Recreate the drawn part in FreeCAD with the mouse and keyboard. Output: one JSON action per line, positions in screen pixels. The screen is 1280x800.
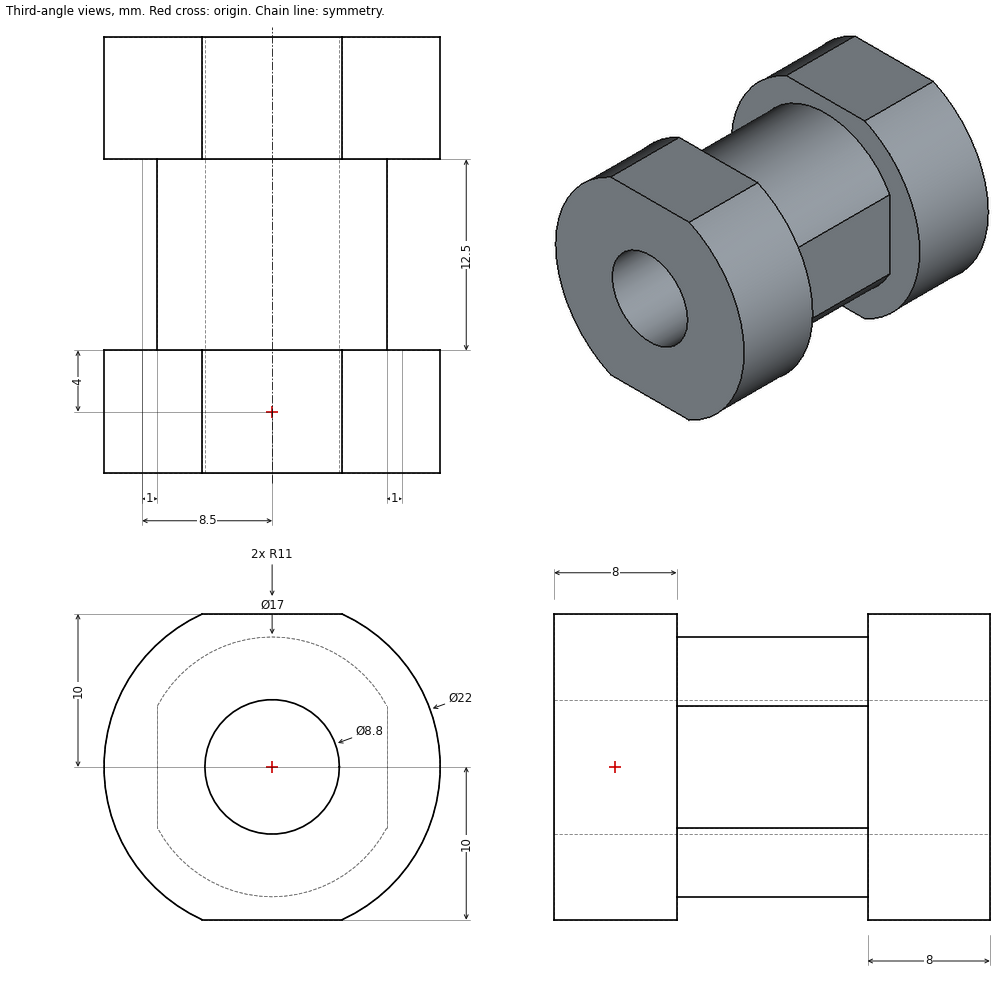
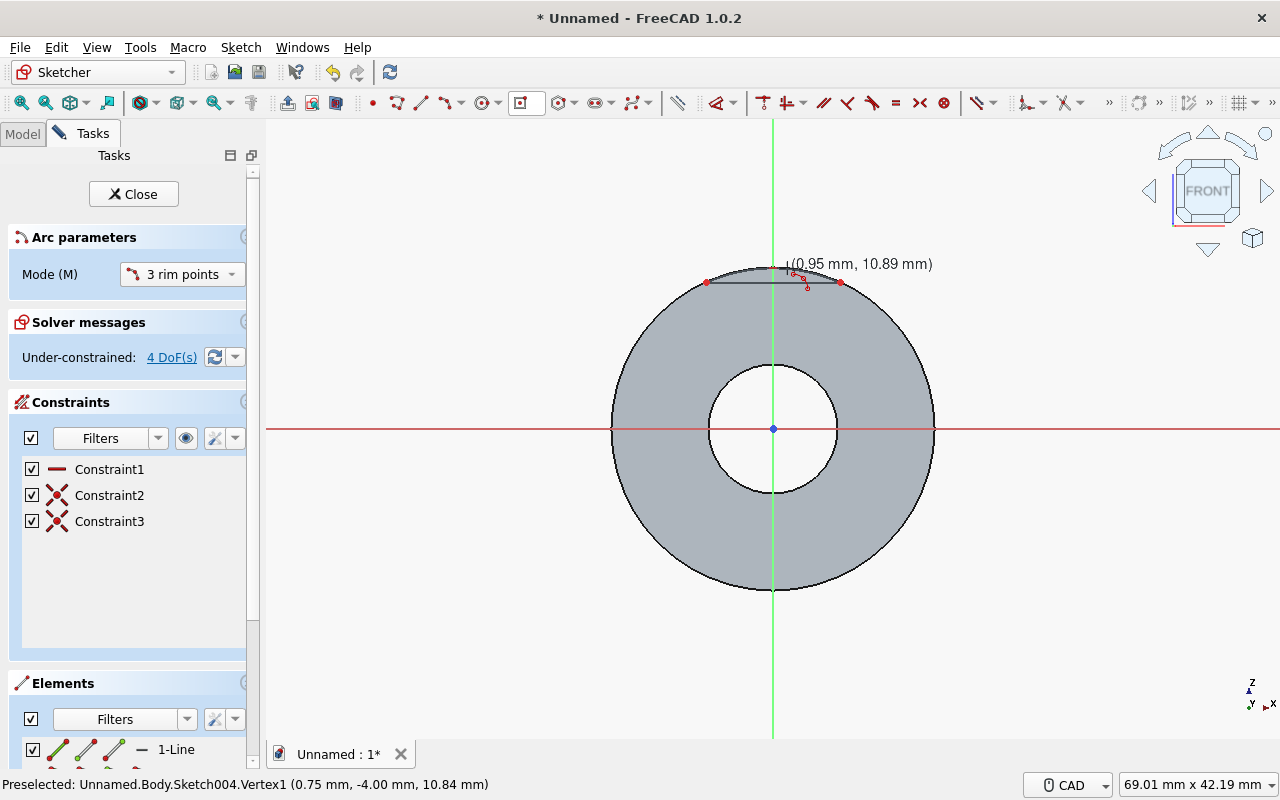
{"action": "left_click", "coordinate": [422, 104]}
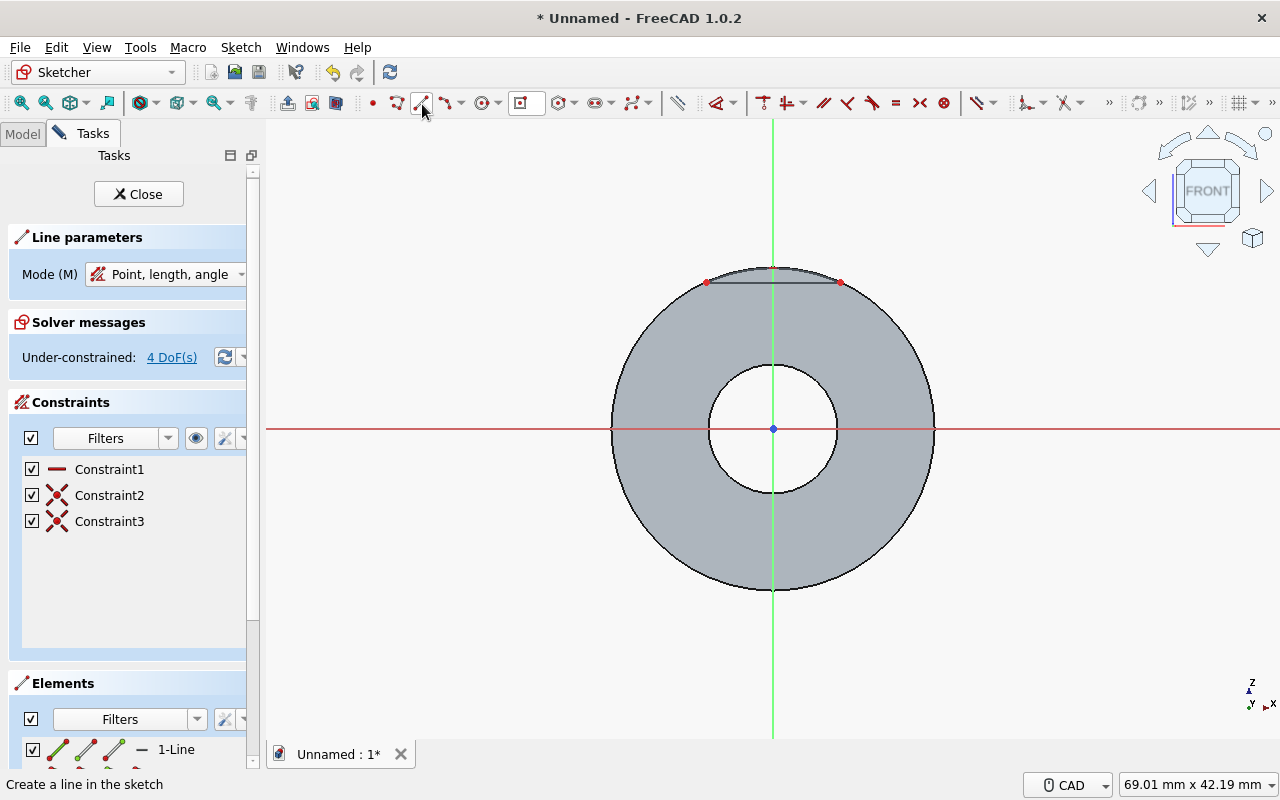
{"action": "left_click", "coordinate": [840, 576]}
{"action": "left_click", "coordinate": [706, 576]}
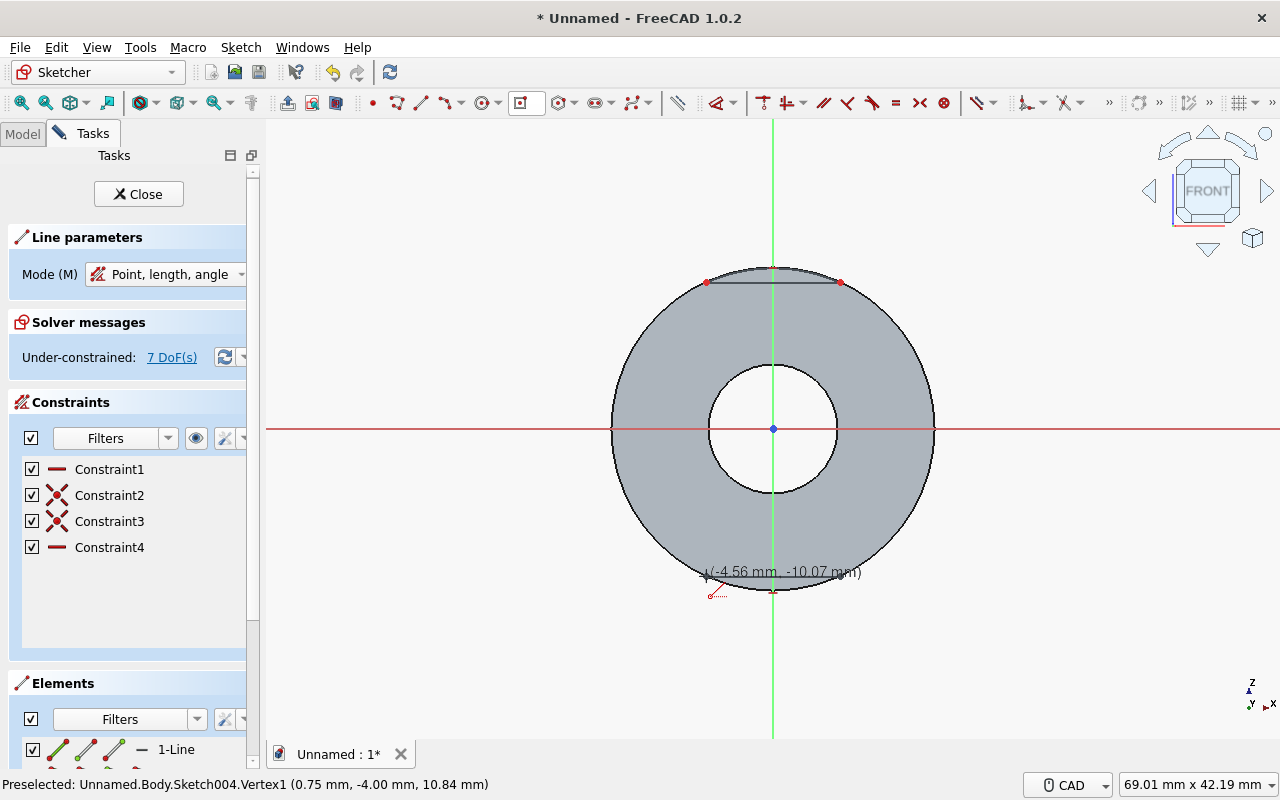
{"action": "left_click", "coordinate": [446, 104]}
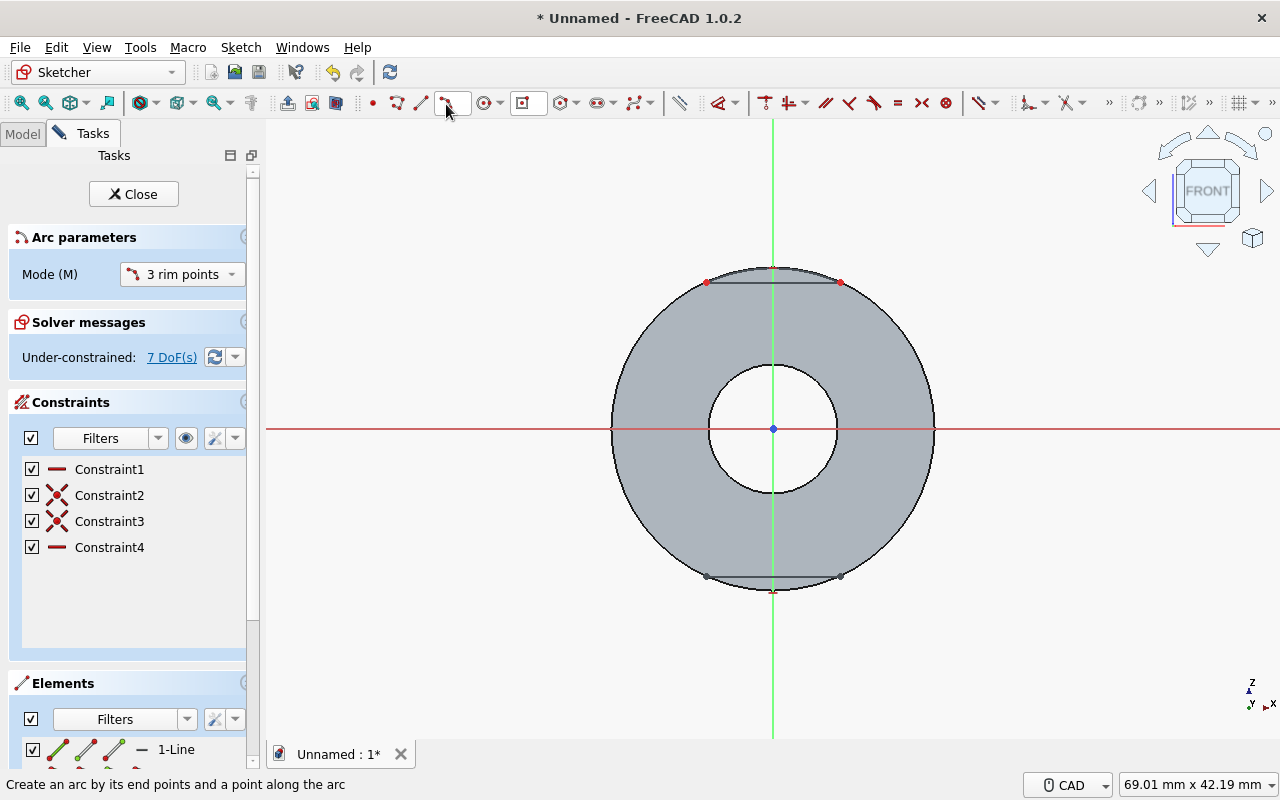
{"action": "left_click", "coordinate": [706, 577]}
{"action": "left_click", "coordinate": [840, 577]}
{"action": "left_click", "coordinate": [787, 590]}
{"action": "key", "text": "Escape"}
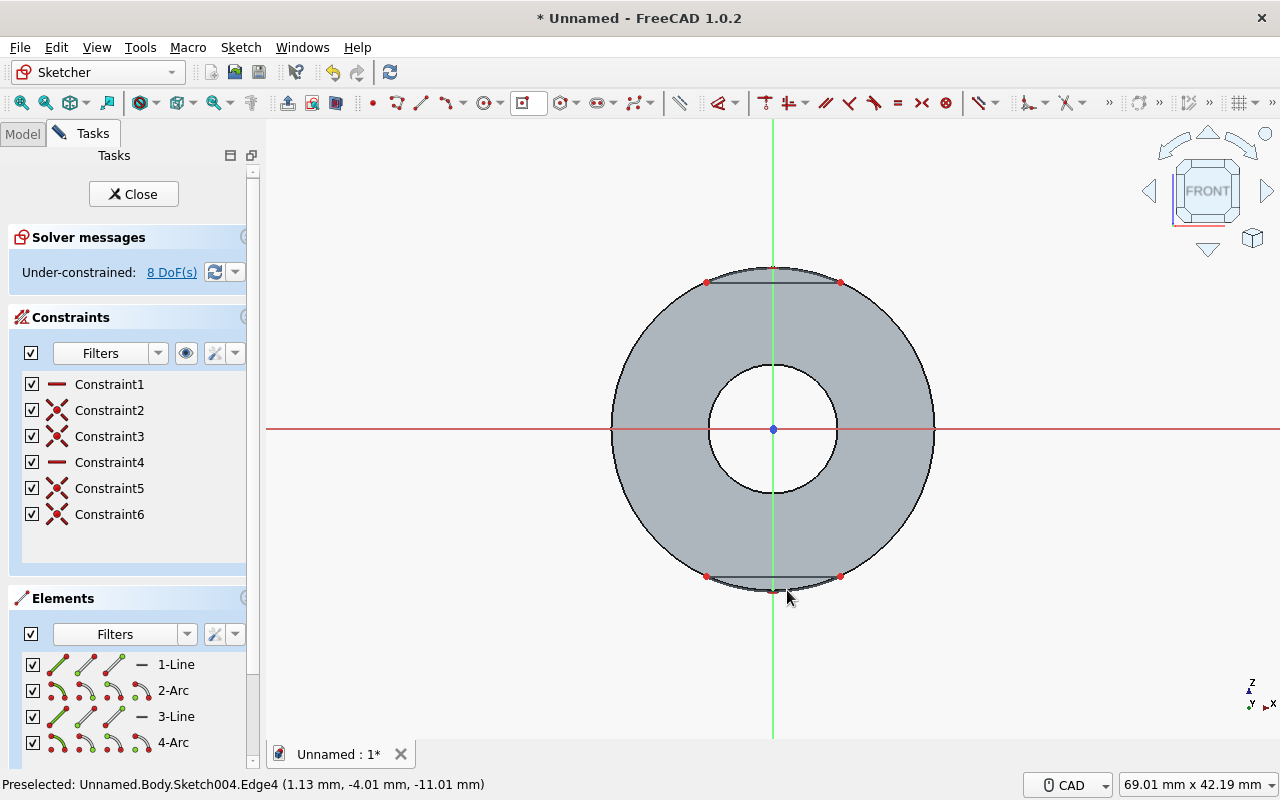
{"action": "left_click", "coordinate": [801, 271]}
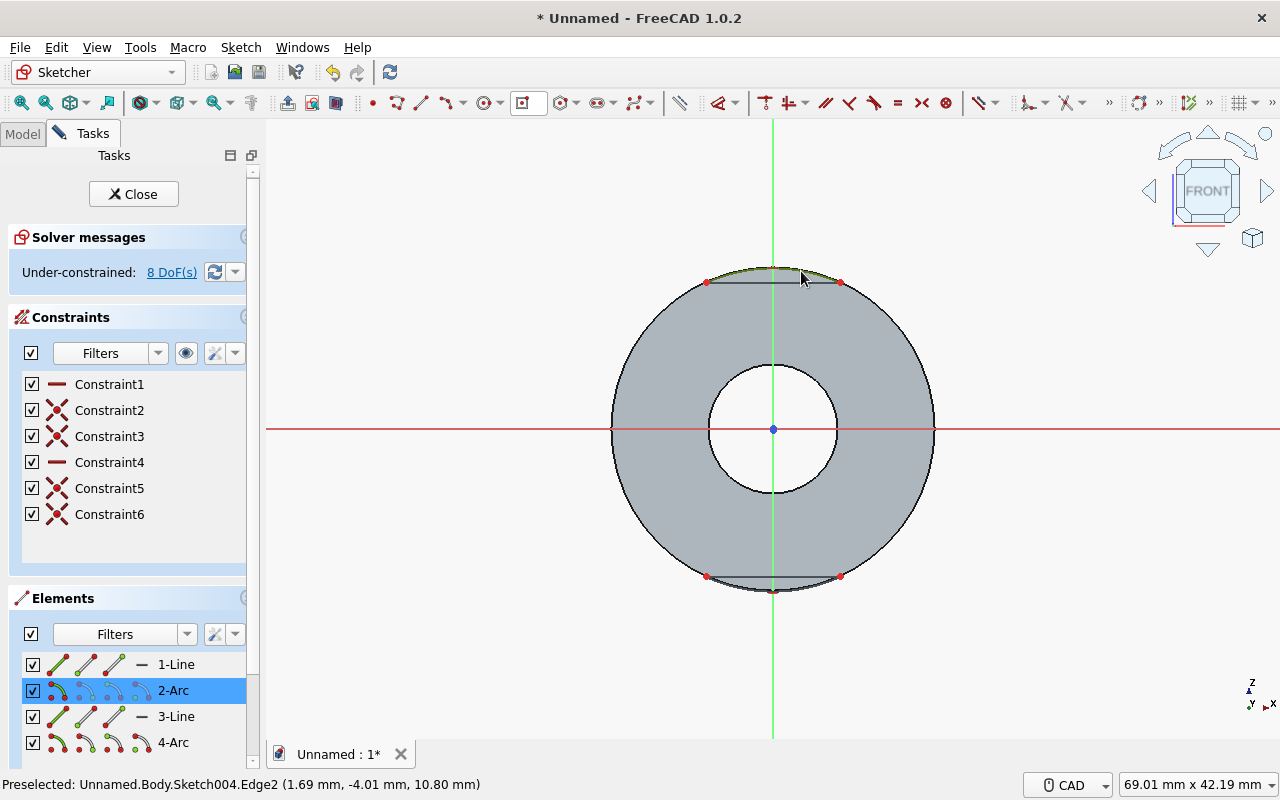
{"action": "left_click", "coordinate": [745, 589]}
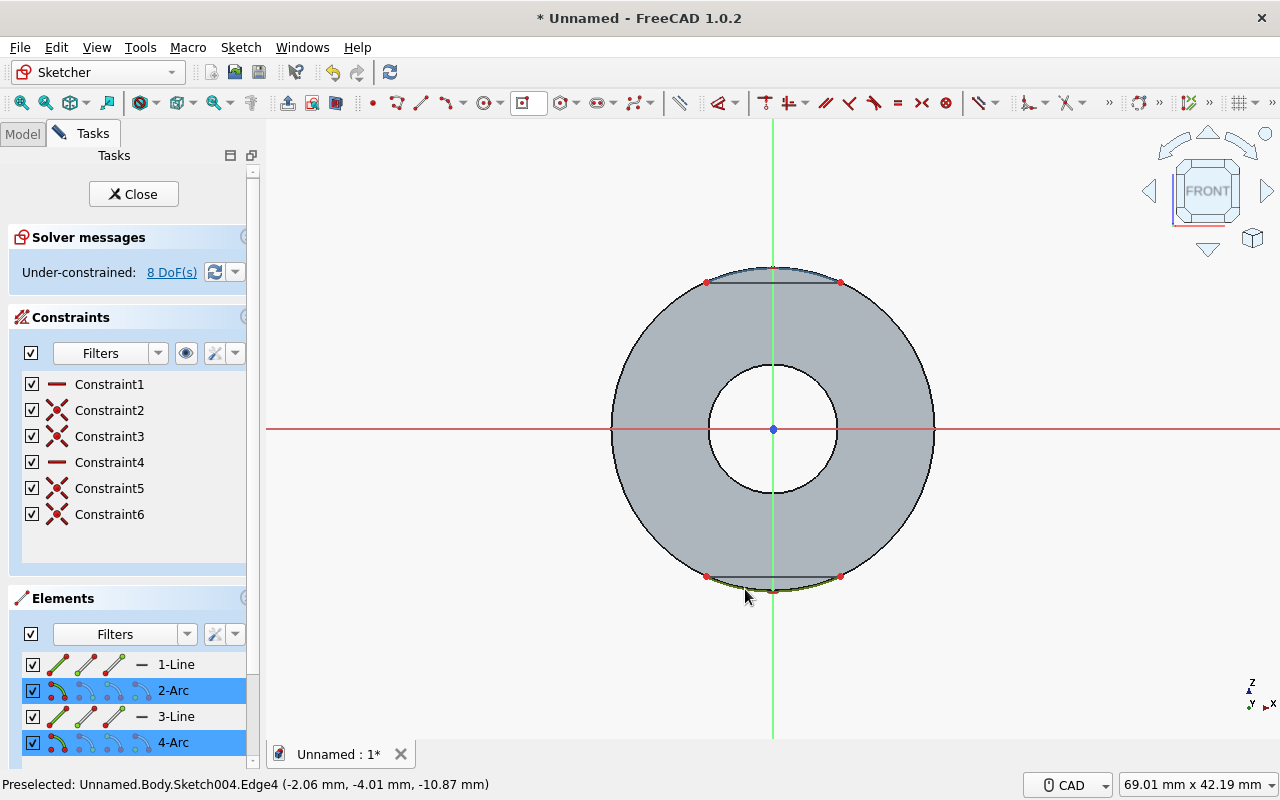
{"action": "left_click", "coordinate": [766, 104]}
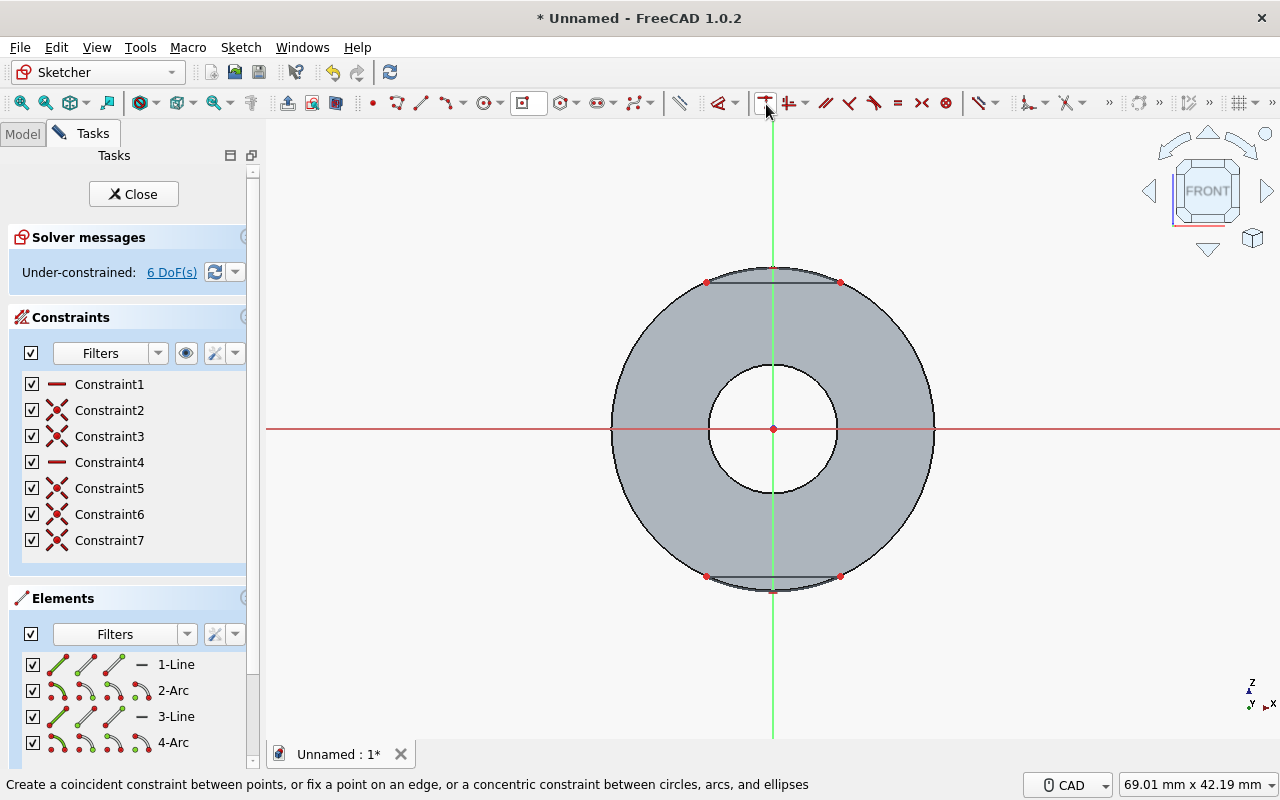
{"action": "left_click_drag", "start_coordinate": [763, 419], "coordinate": [783, 439]}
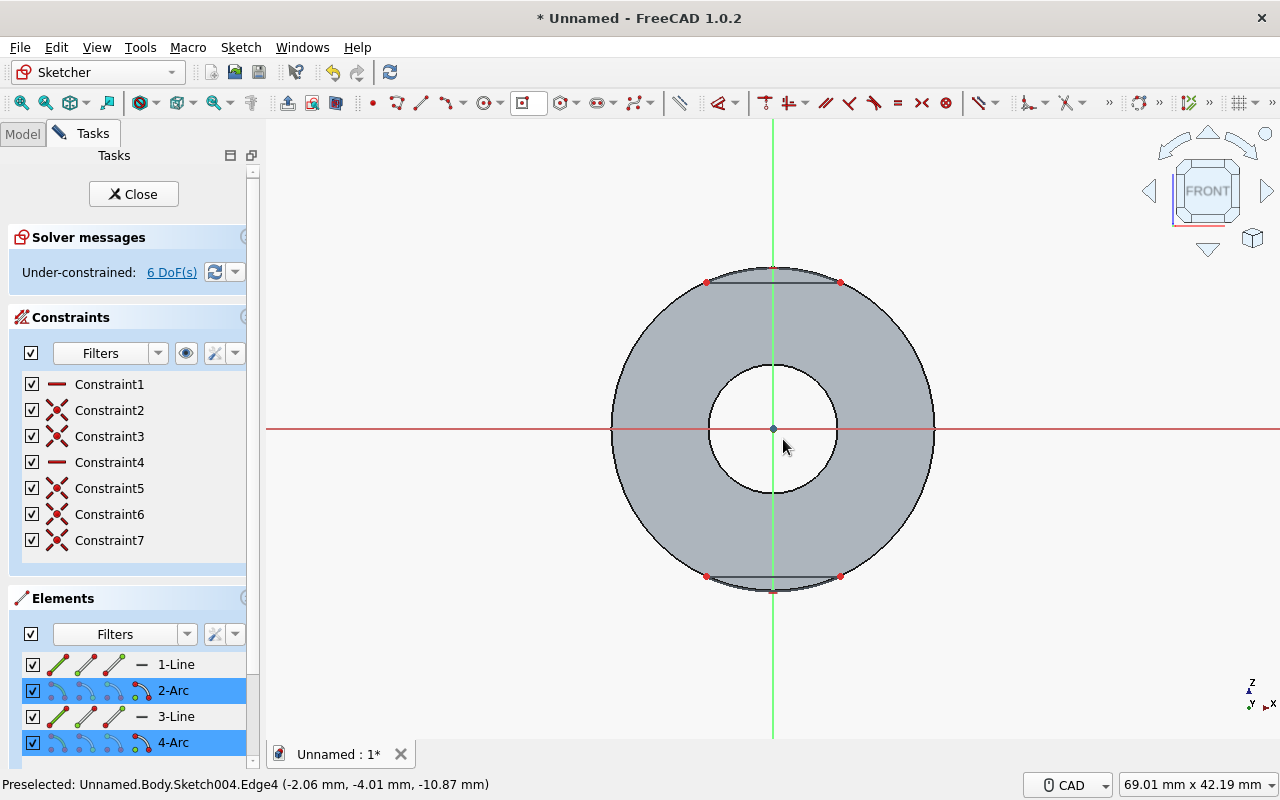
{"action": "left_click", "coordinate": [766, 104]}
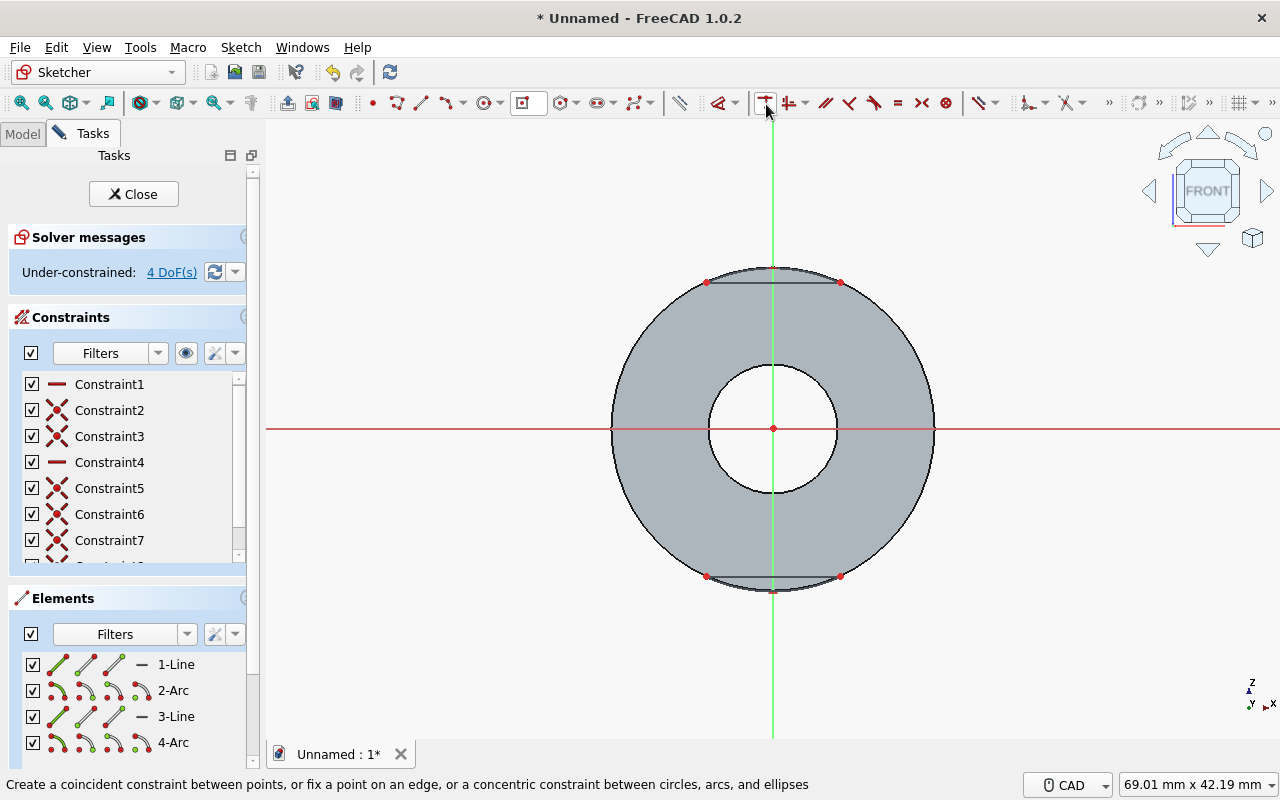
{"action": "left_click", "coordinate": [801, 271]}